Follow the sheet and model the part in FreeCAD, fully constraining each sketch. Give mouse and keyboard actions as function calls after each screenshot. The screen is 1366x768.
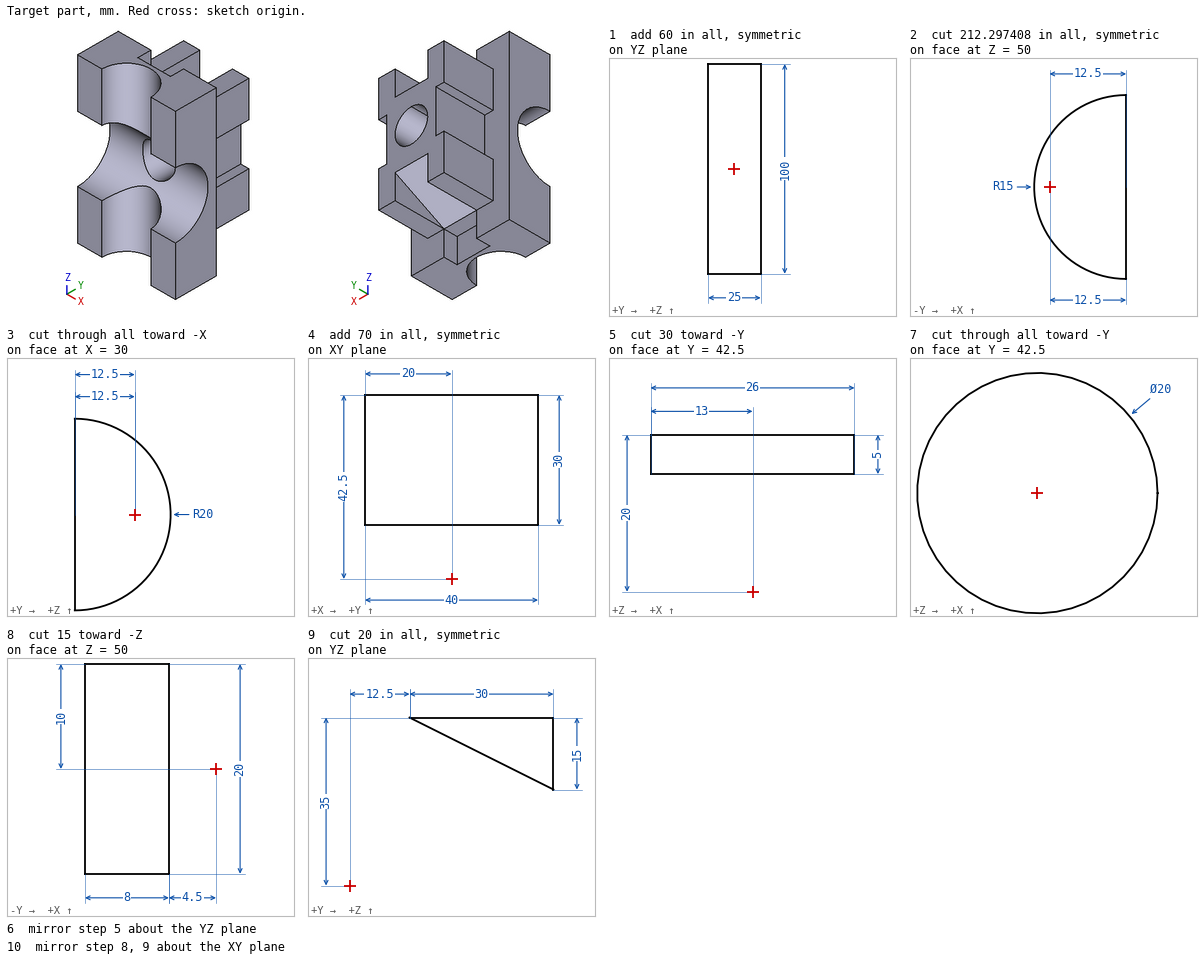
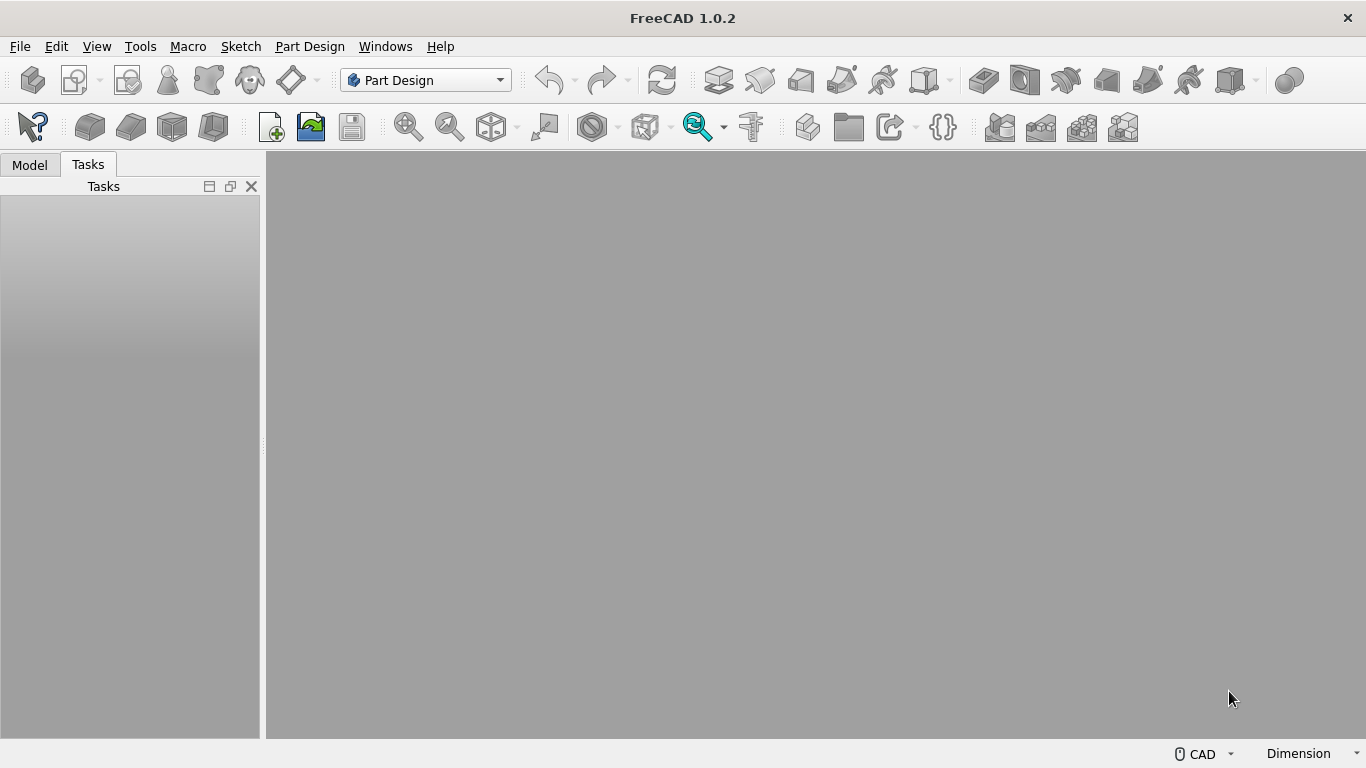
key(ctrl+n)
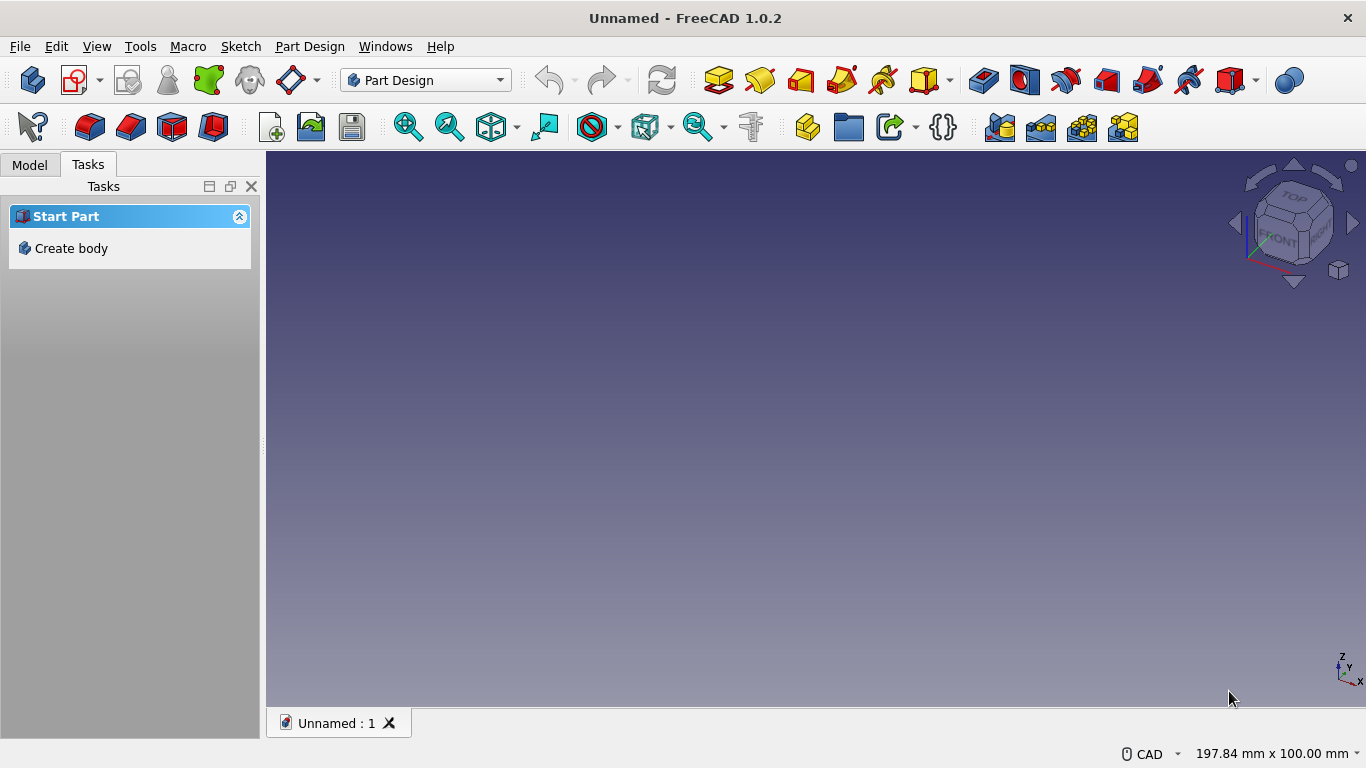
click(74, 80)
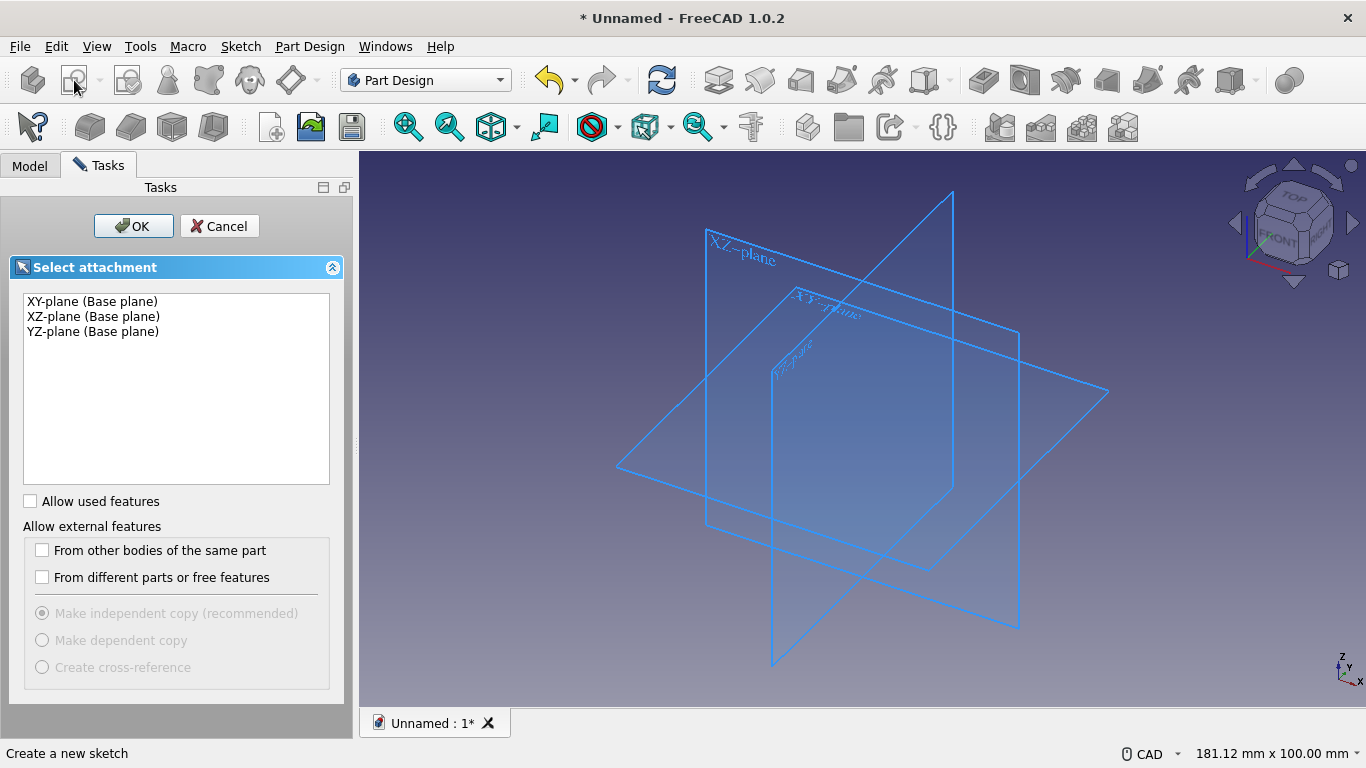
click(84, 332)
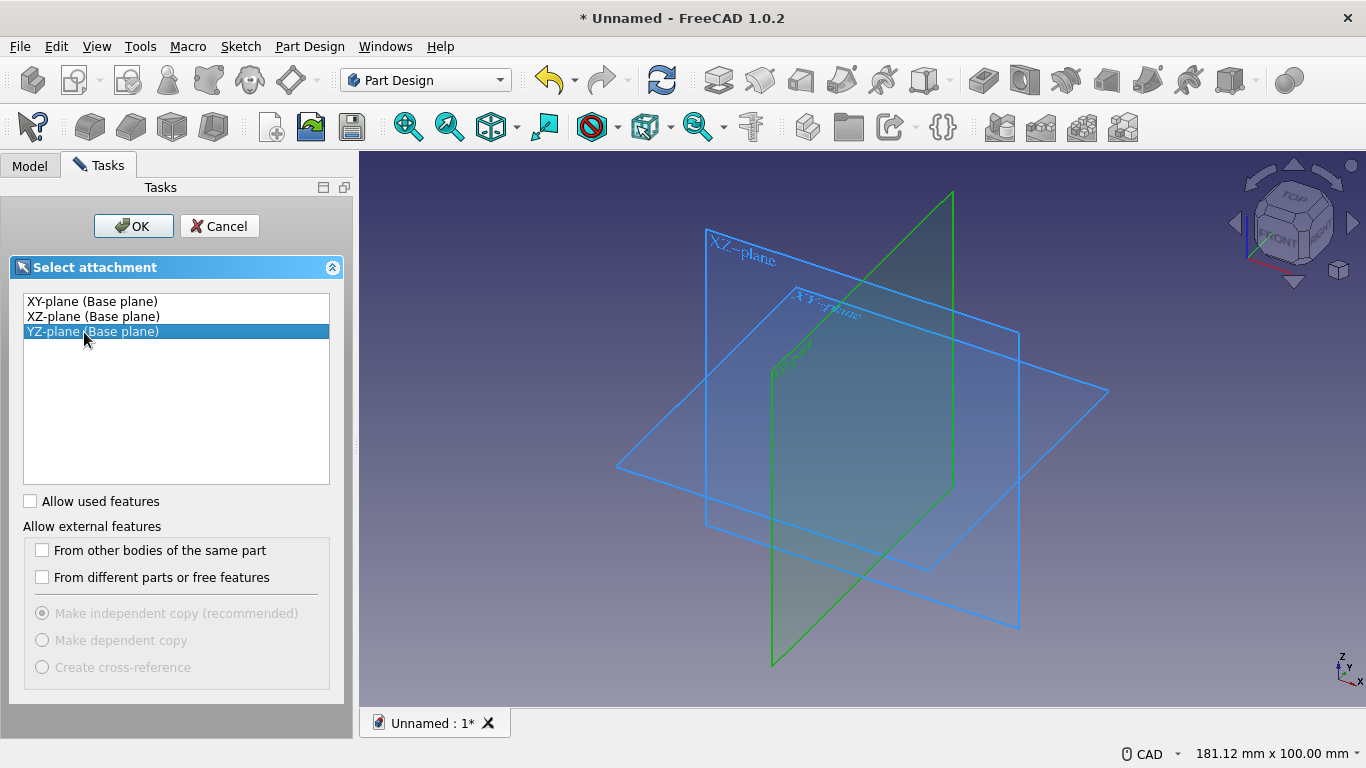
click(134, 226)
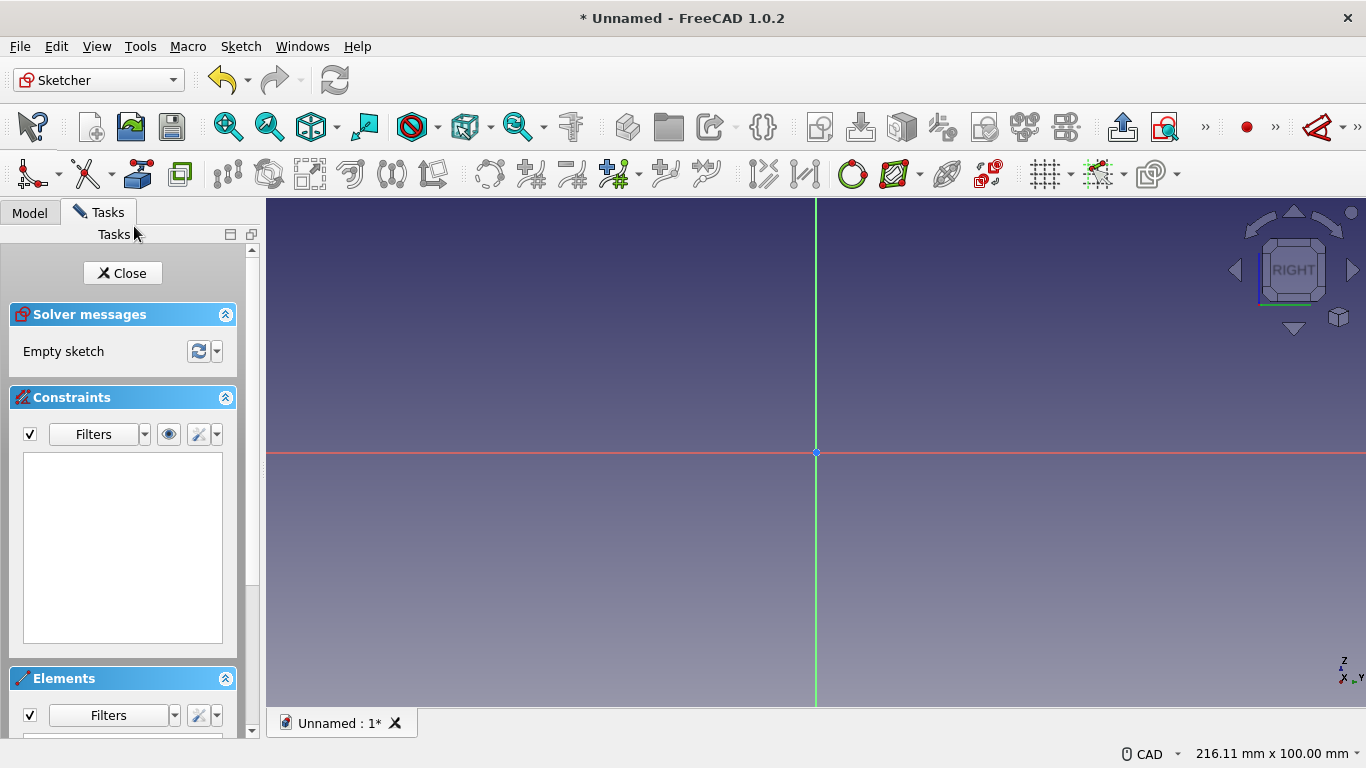
scroll(608, 453, down, 2)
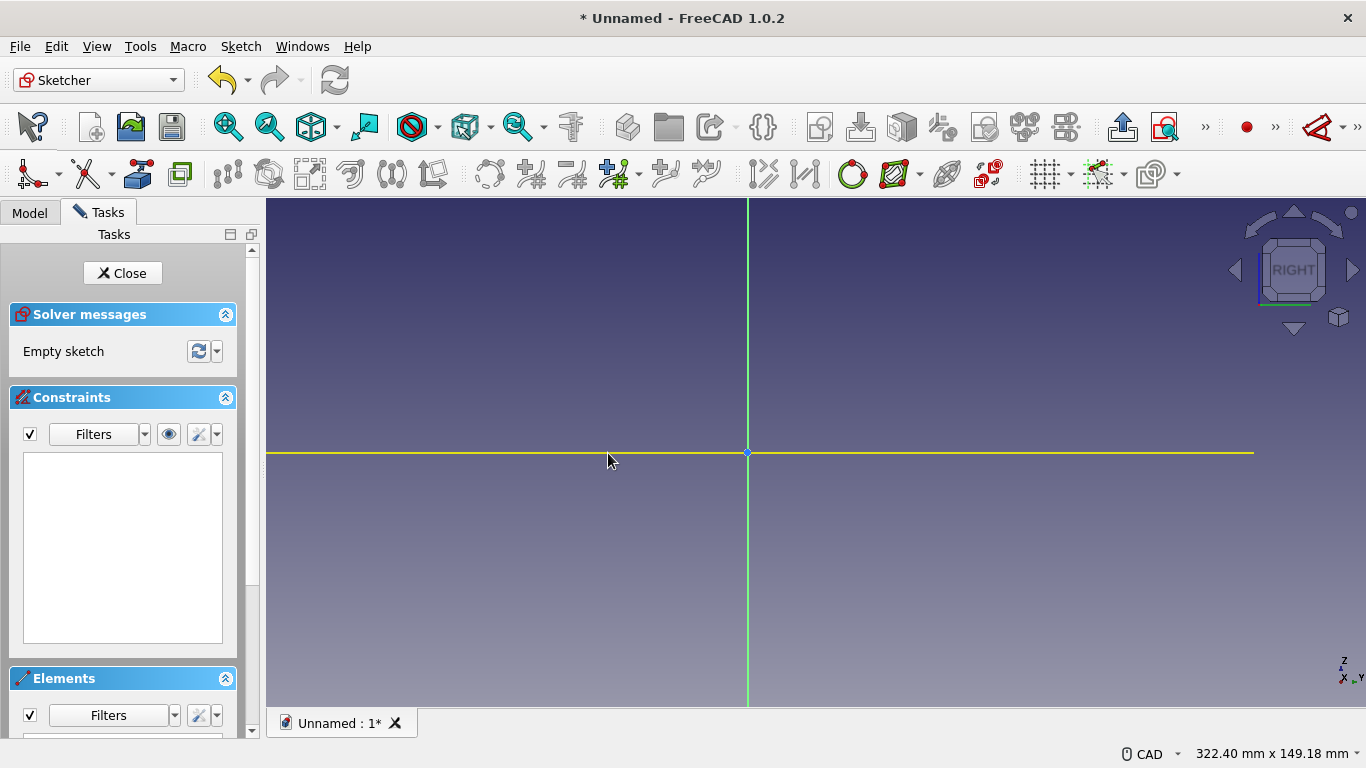
key(g)
key(v)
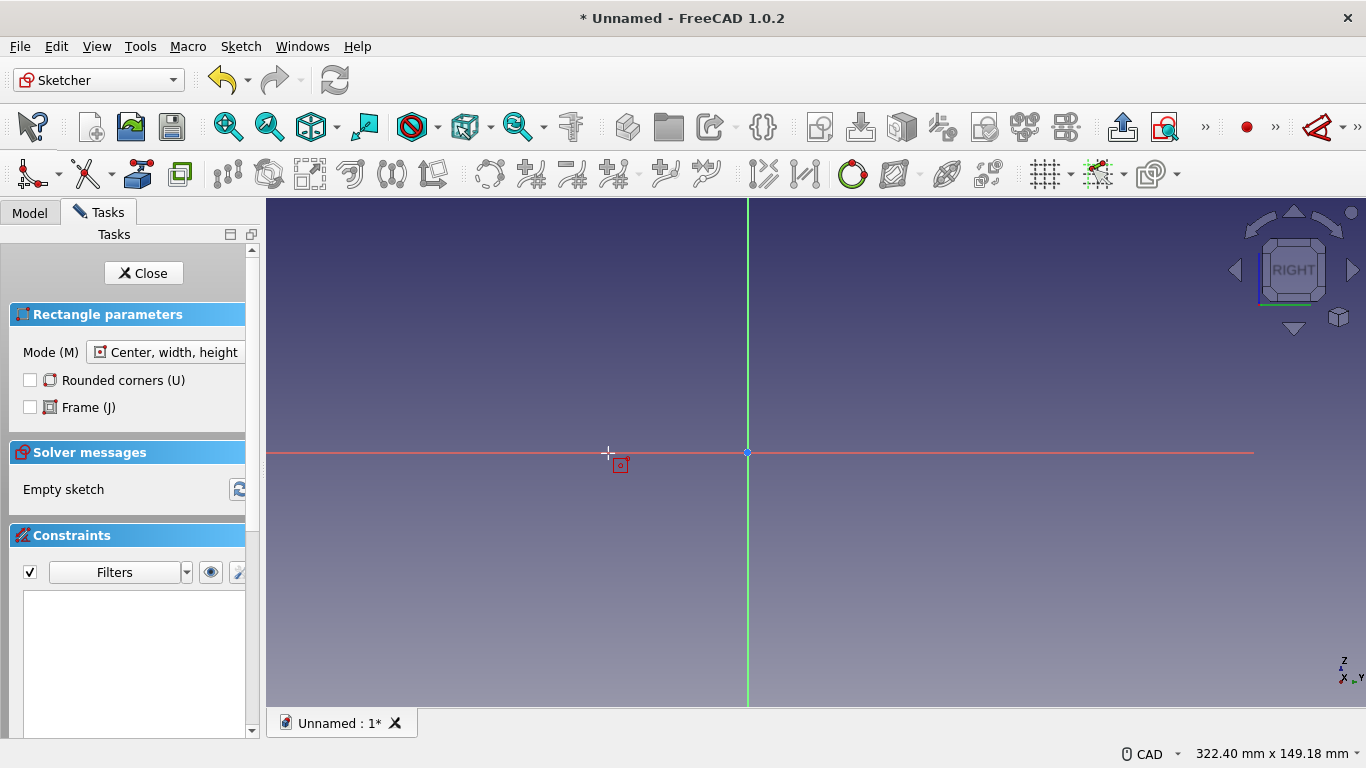
click(748, 453)
move(790, 282)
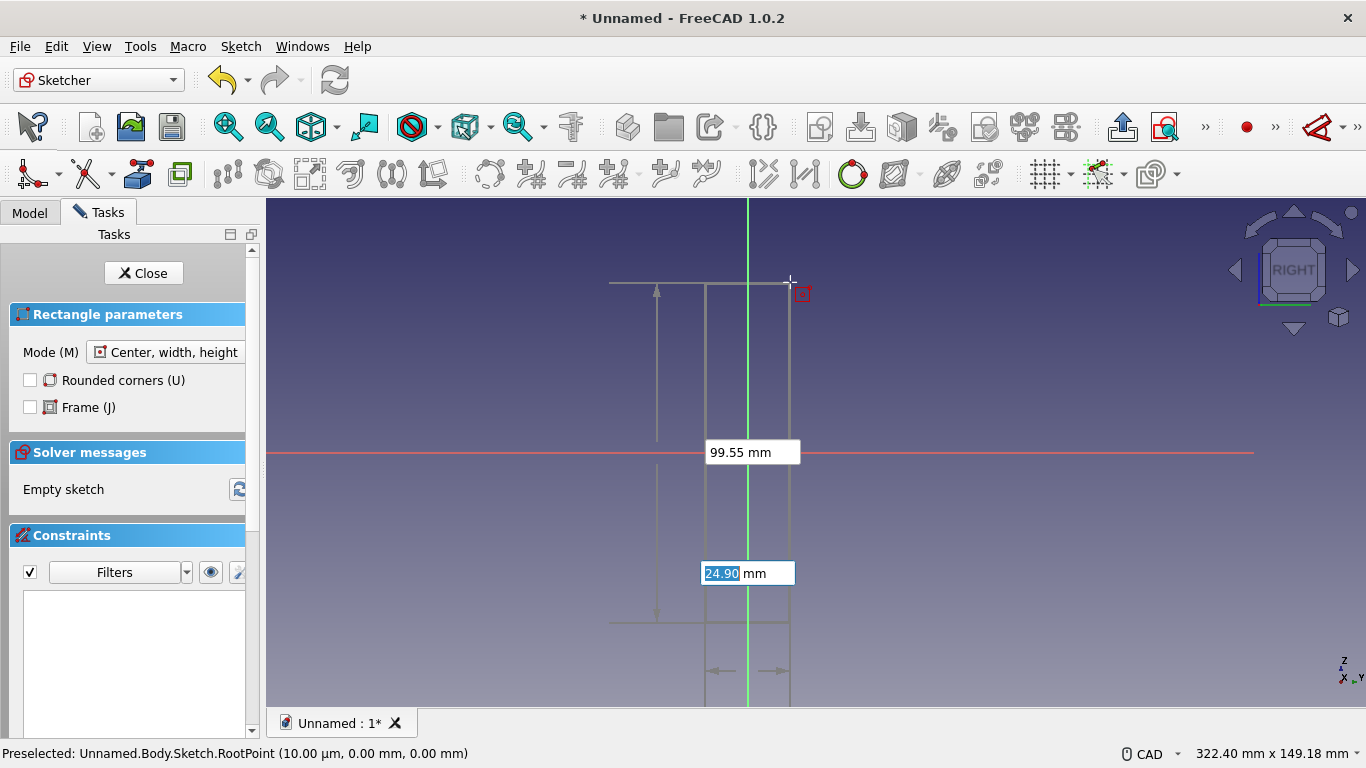
text(25)
key(Tab)
text(100)
key(Return)
key(Escape)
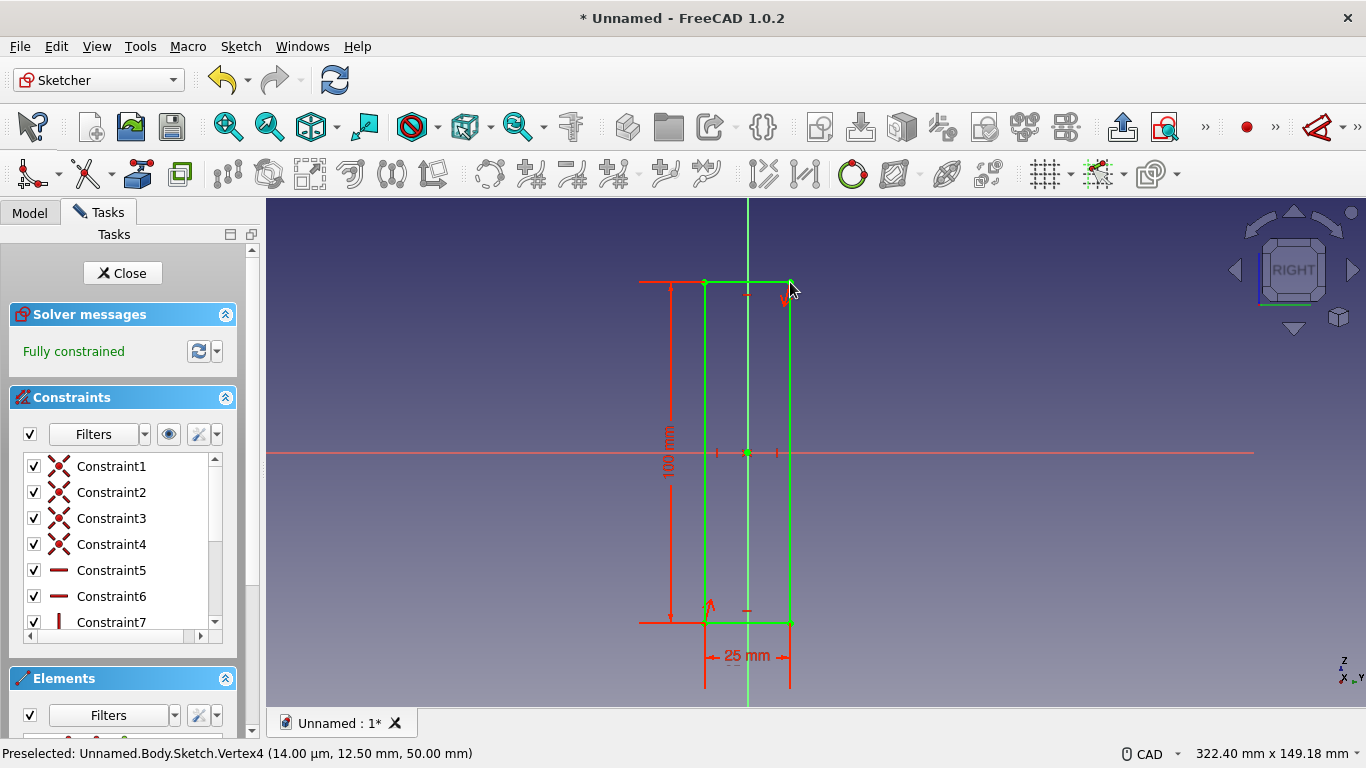
click(123, 273)